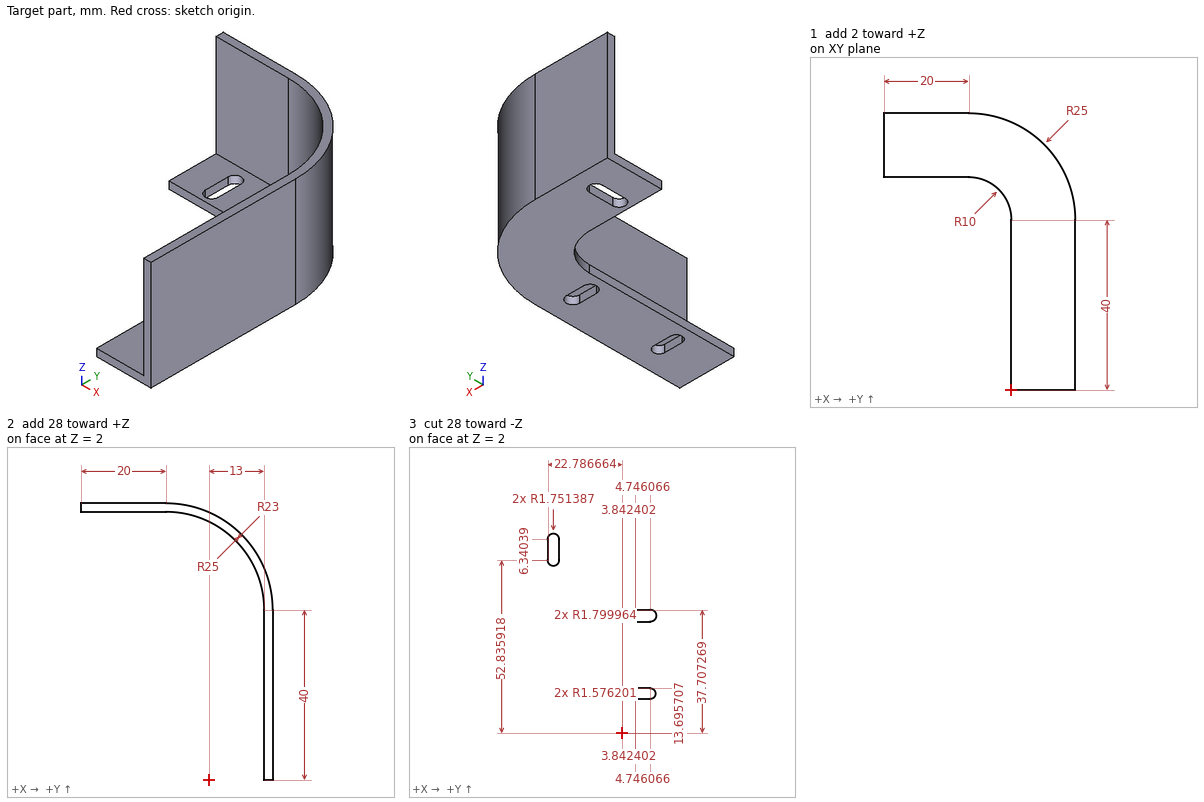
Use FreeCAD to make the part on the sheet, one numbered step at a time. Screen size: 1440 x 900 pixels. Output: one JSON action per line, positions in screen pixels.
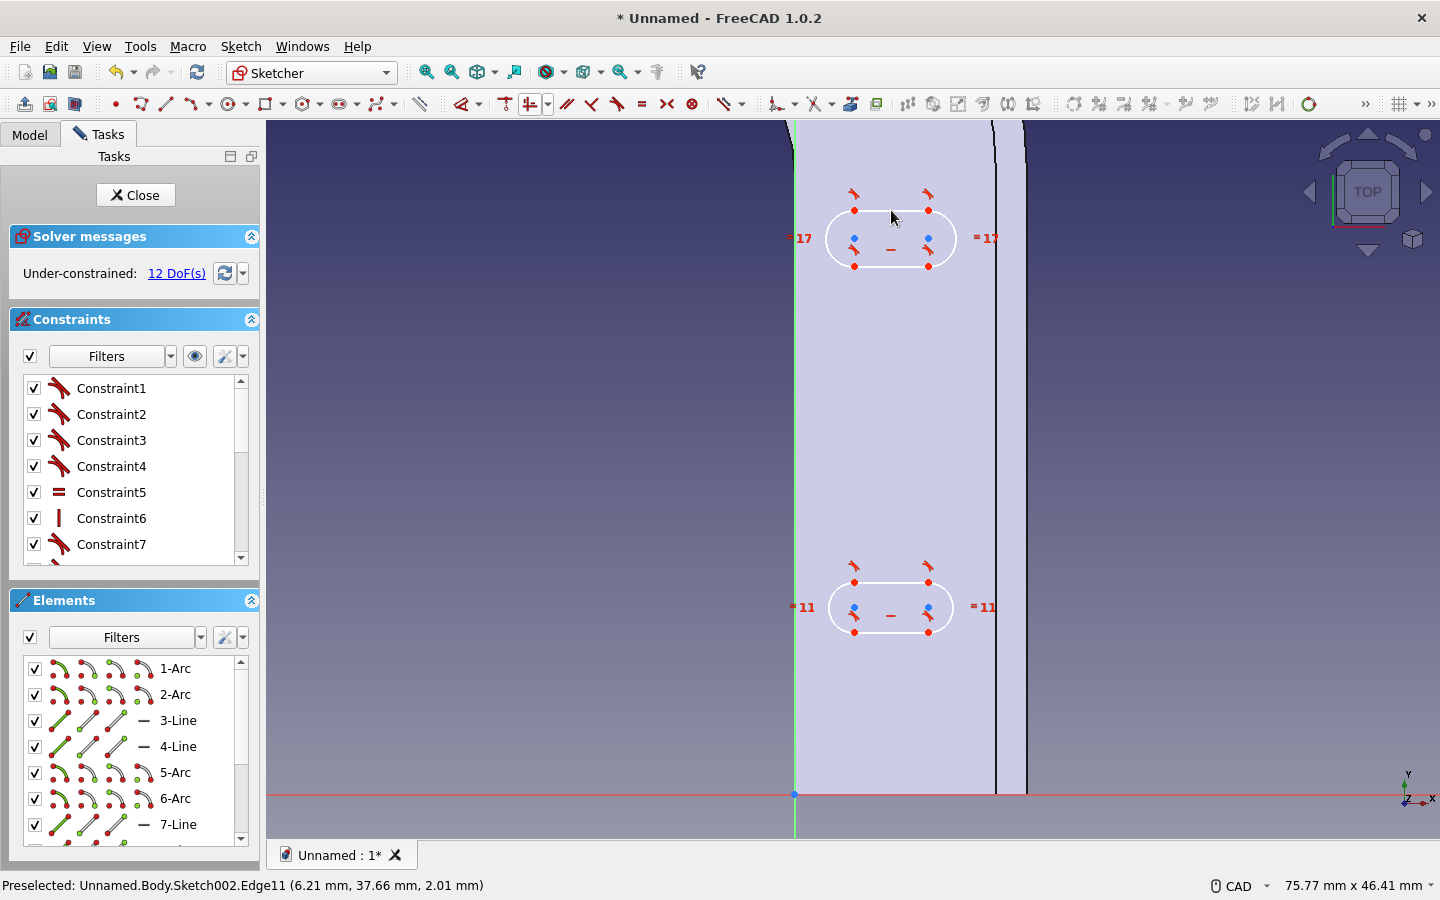
{"action": "key", "text": "d"}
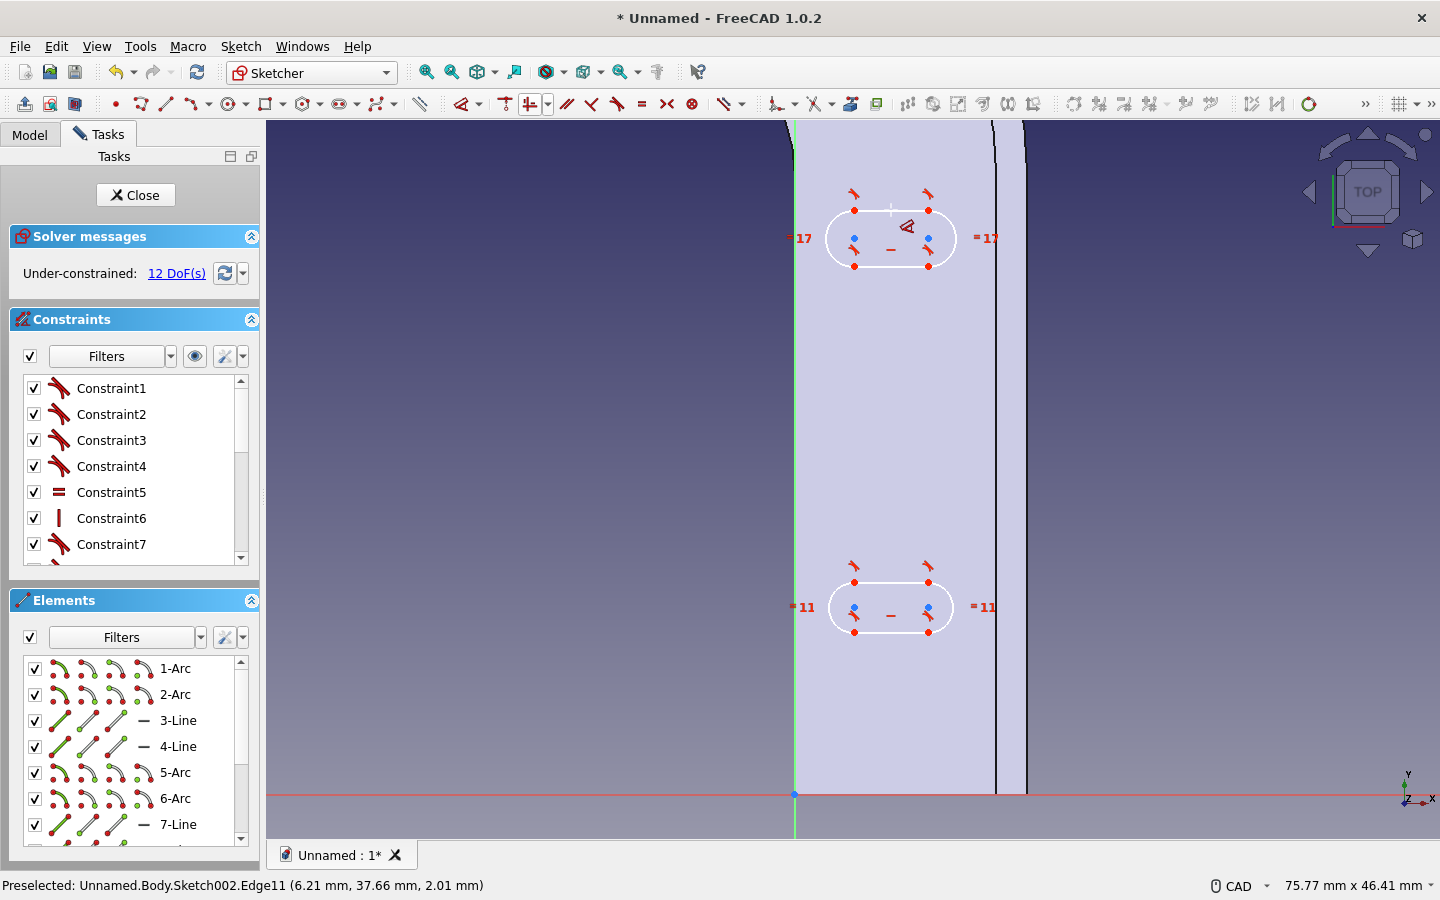
{"action": "scroll", "coordinate": [854, 608], "scroll_direction": "down", "scroll_amount": 4}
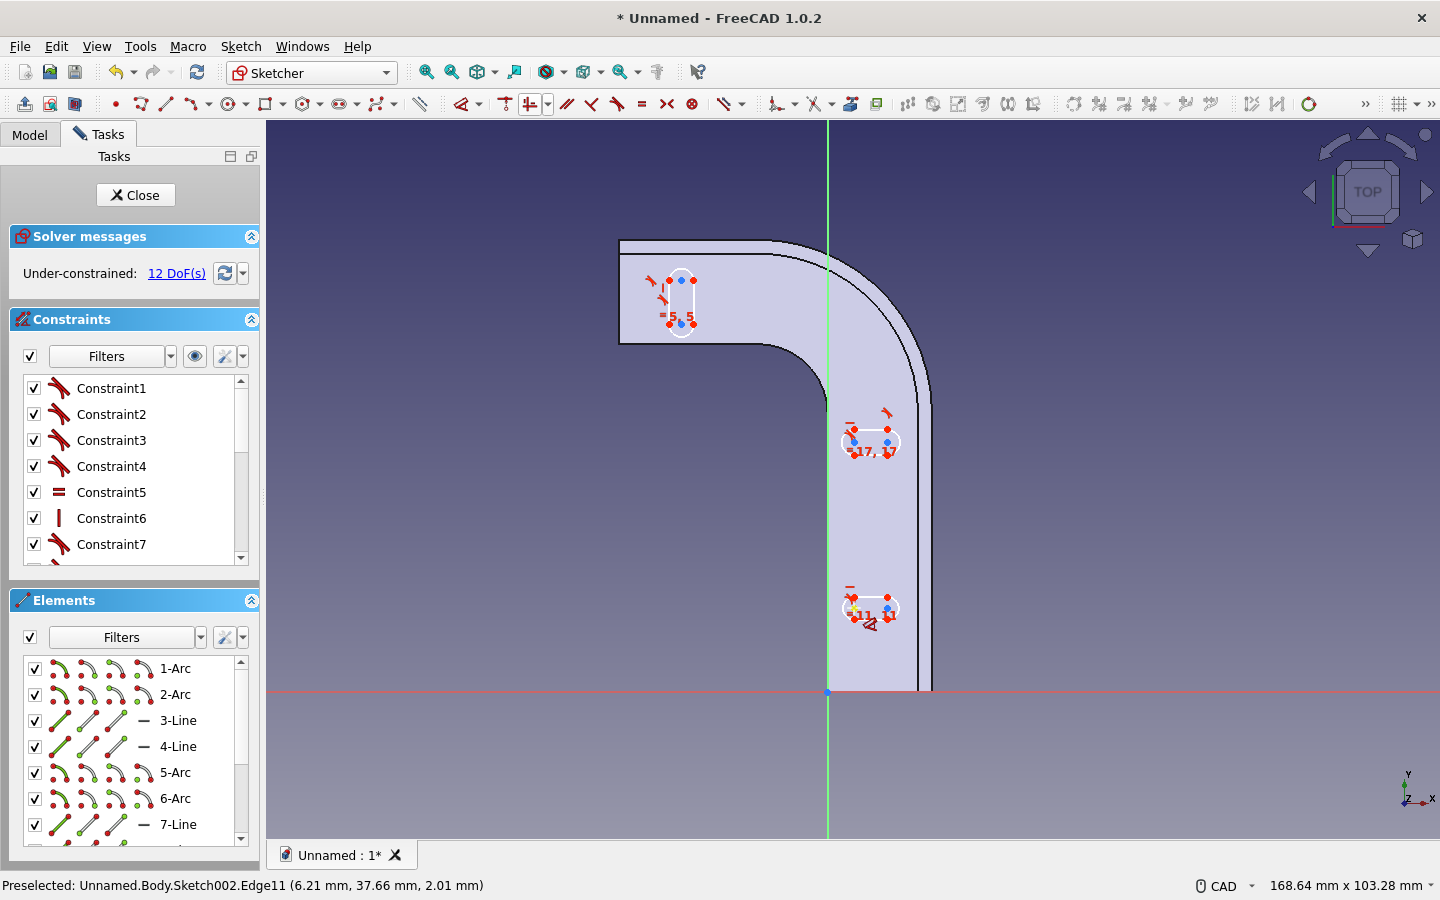
{"action": "scroll", "coordinate": [674, 335], "scroll_direction": "up", "scroll_amount": 6}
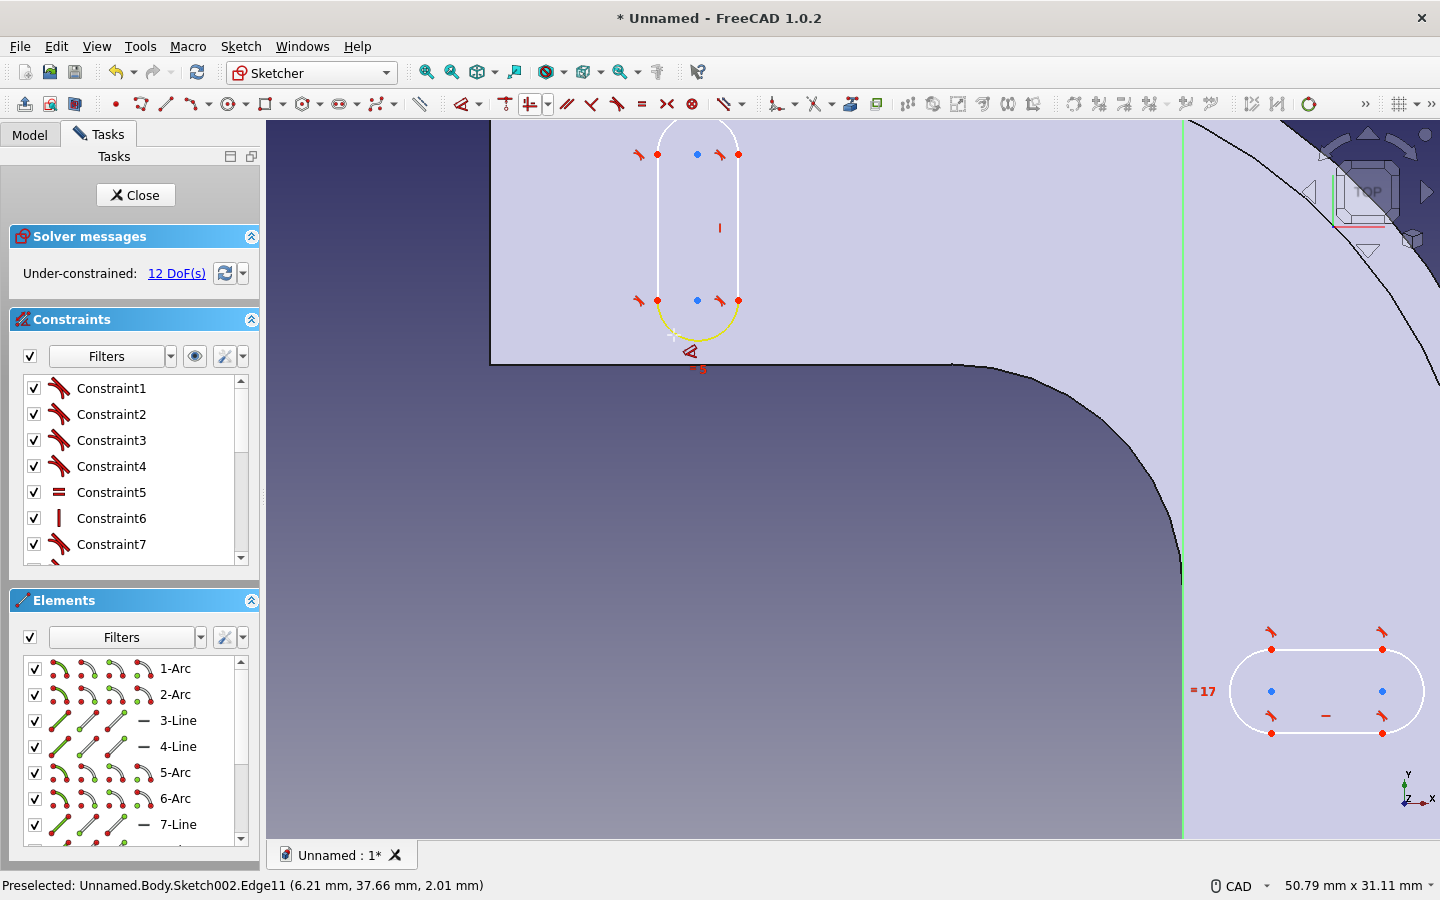
{"action": "left_click", "coordinate": [674, 333]}
{"action": "left_click", "coordinate": [655, 359]}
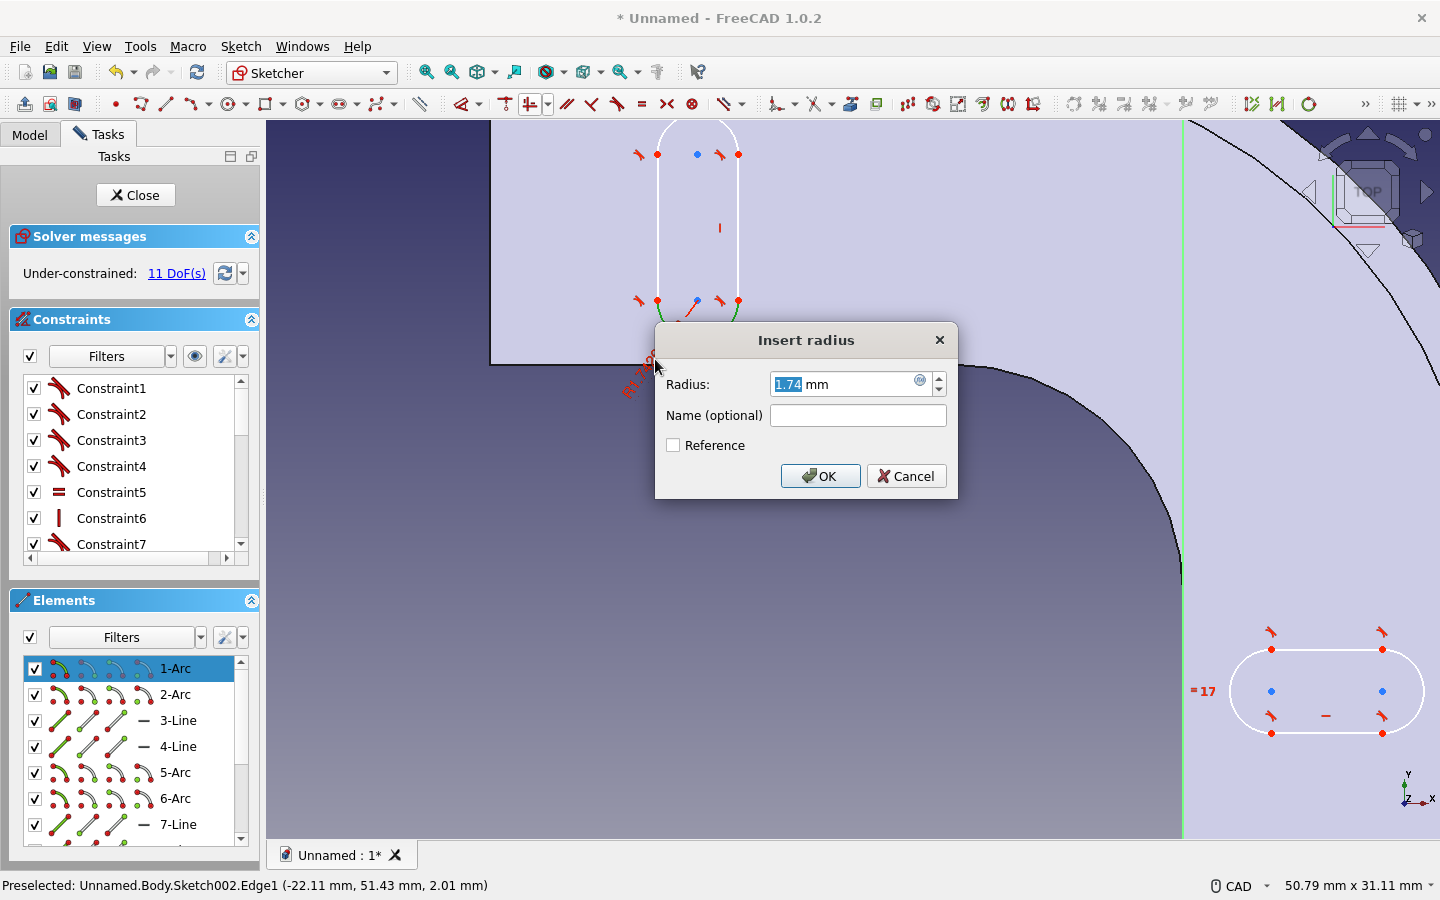
{"action": "type", "text": "1.751387"}
{"action": "key", "text": "Return"}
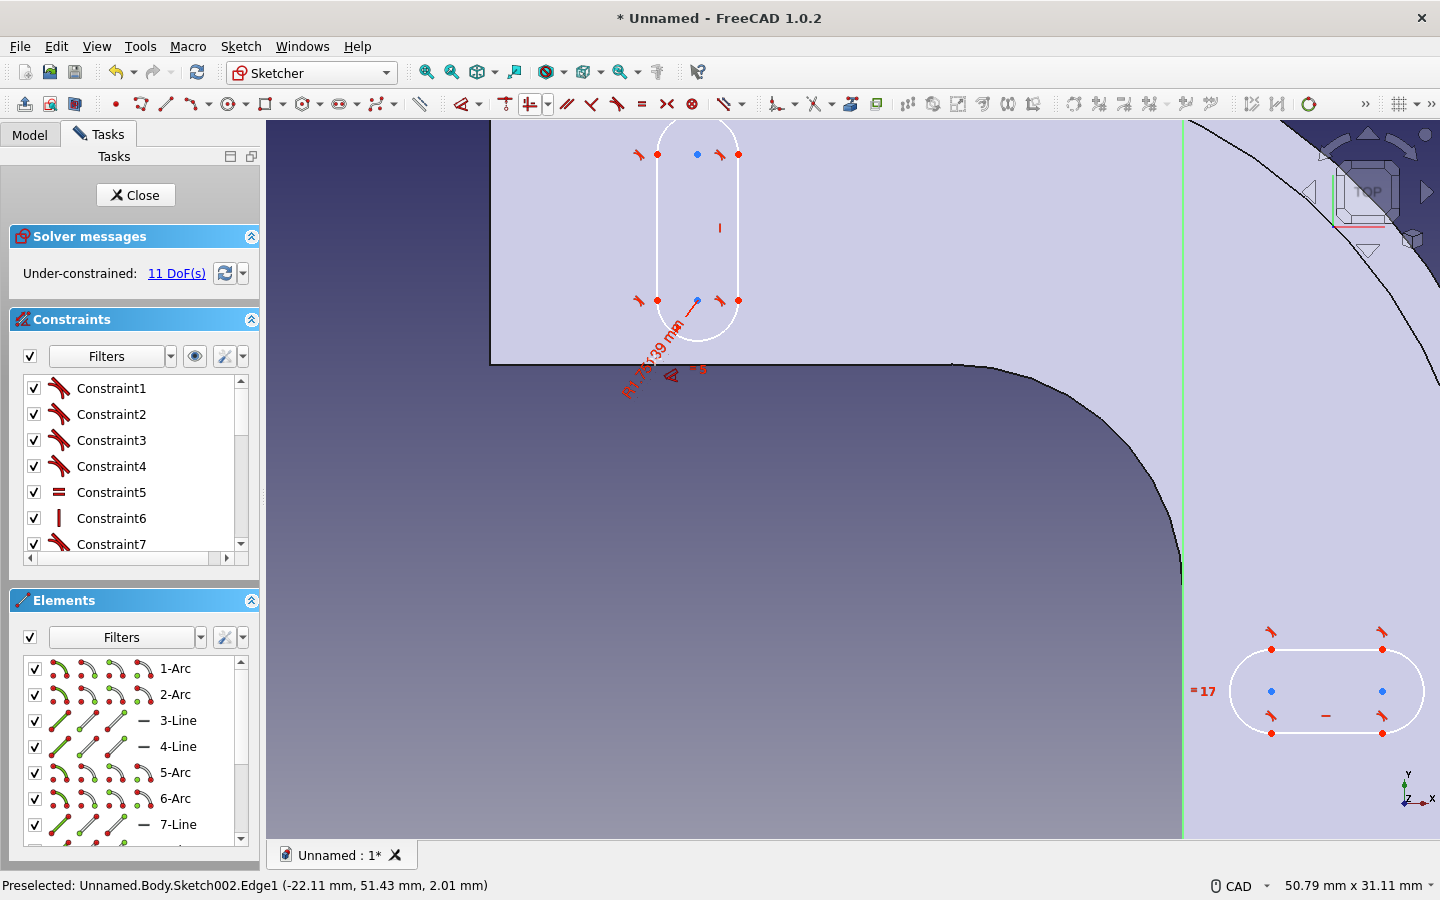
{"action": "scroll", "coordinate": [674, 334], "scroll_direction": "down", "scroll_amount": 6}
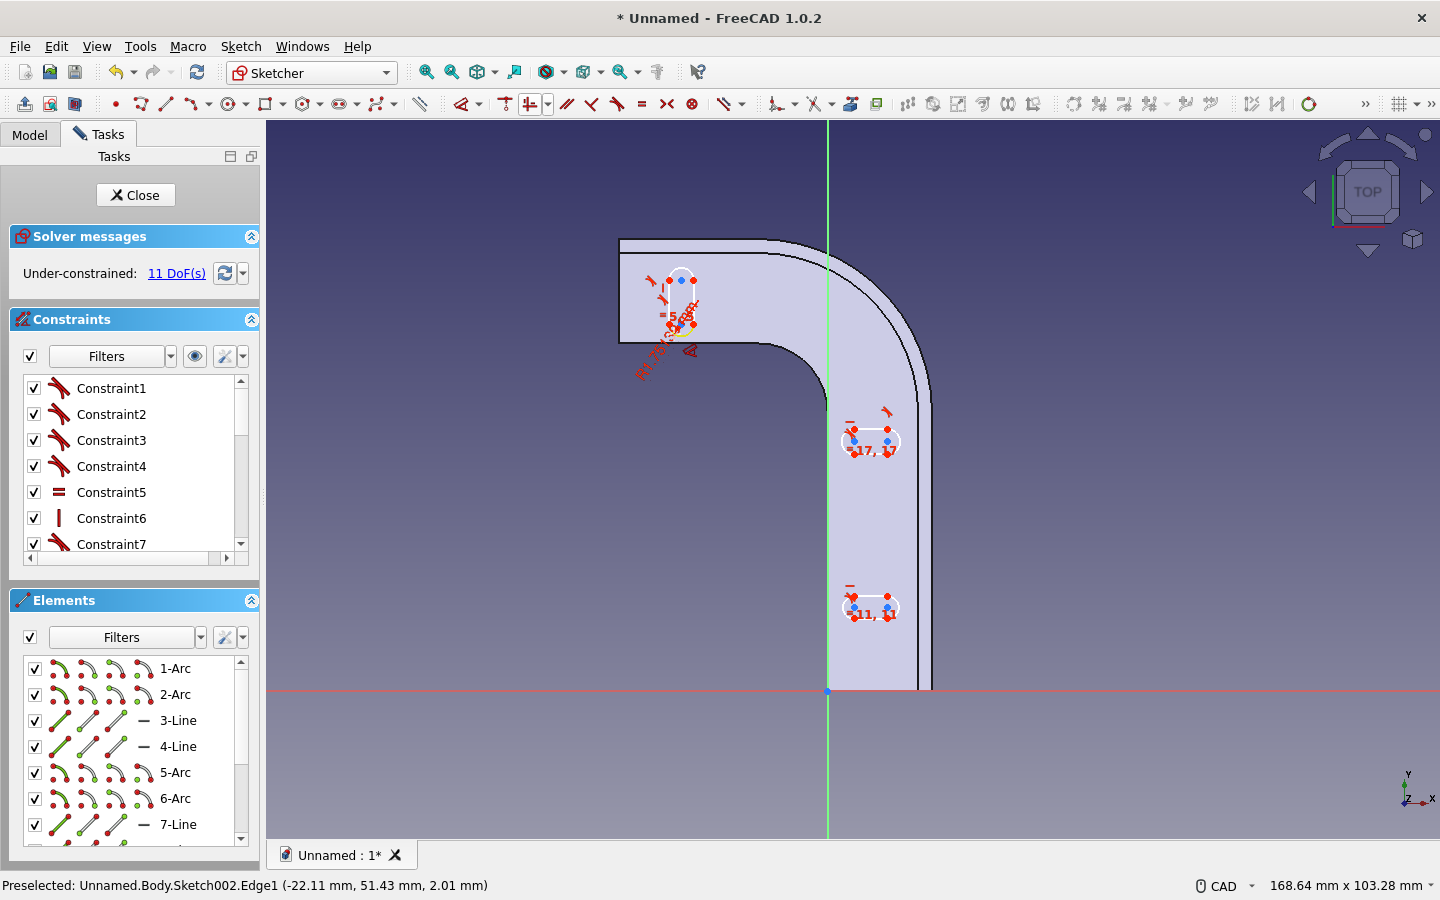
{"action": "scroll", "coordinate": [845, 601], "scroll_direction": "up", "scroll_amount": 7}